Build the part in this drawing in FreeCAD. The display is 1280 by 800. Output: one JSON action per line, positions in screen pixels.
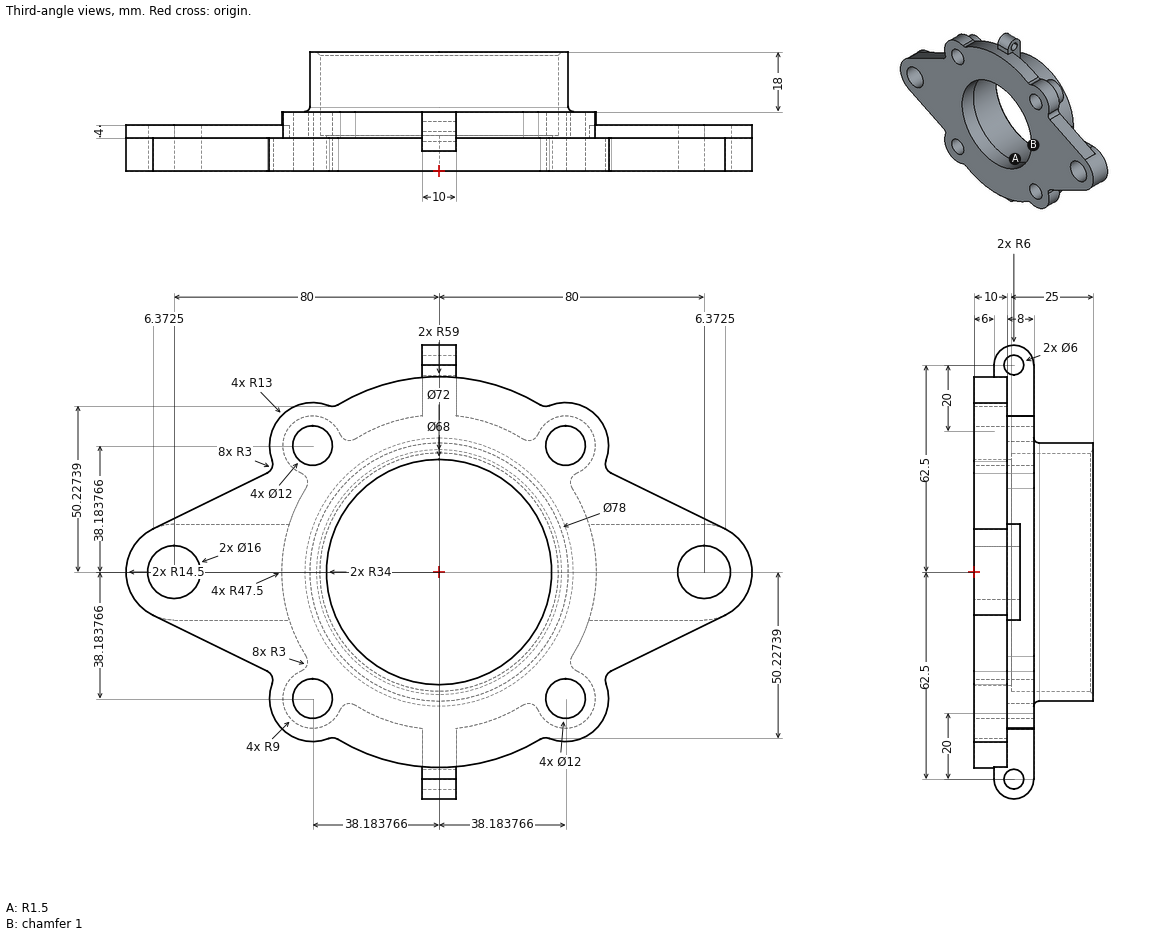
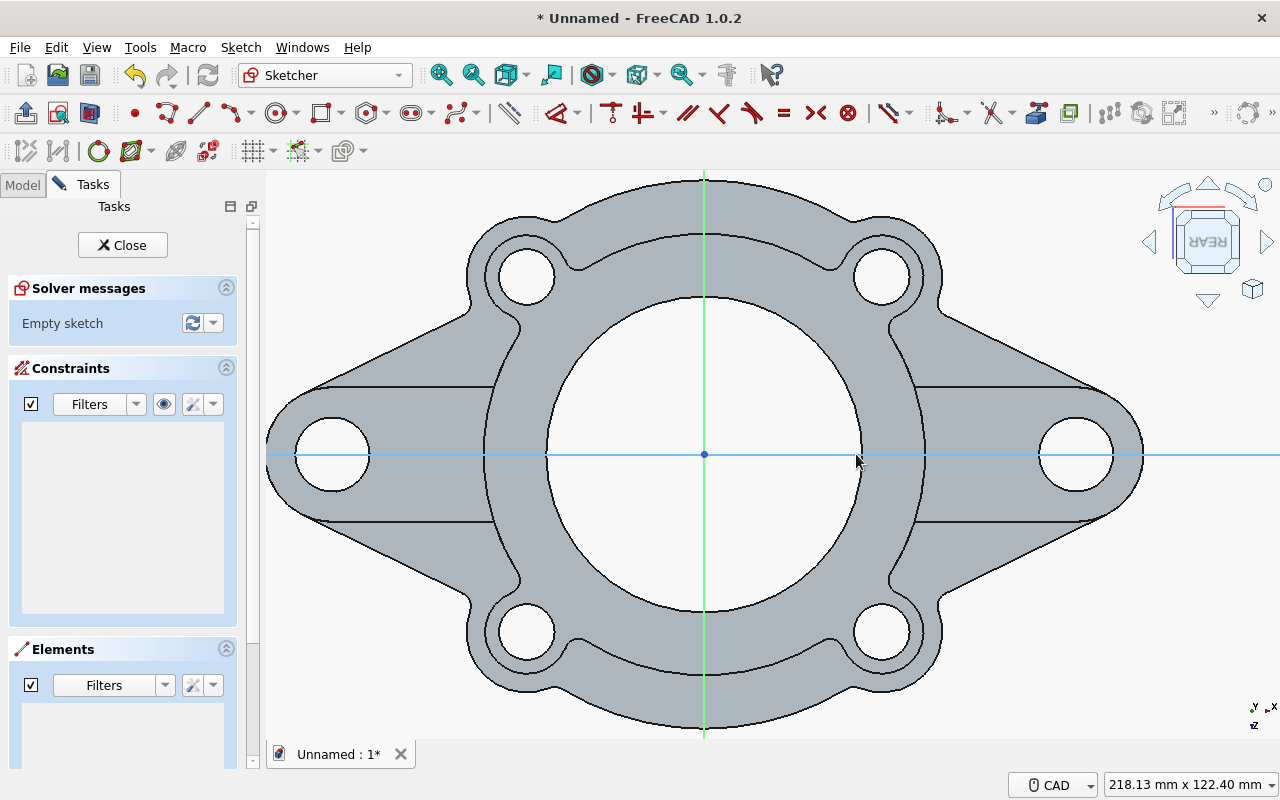
{"action": "left_click", "coordinate": [276, 114]}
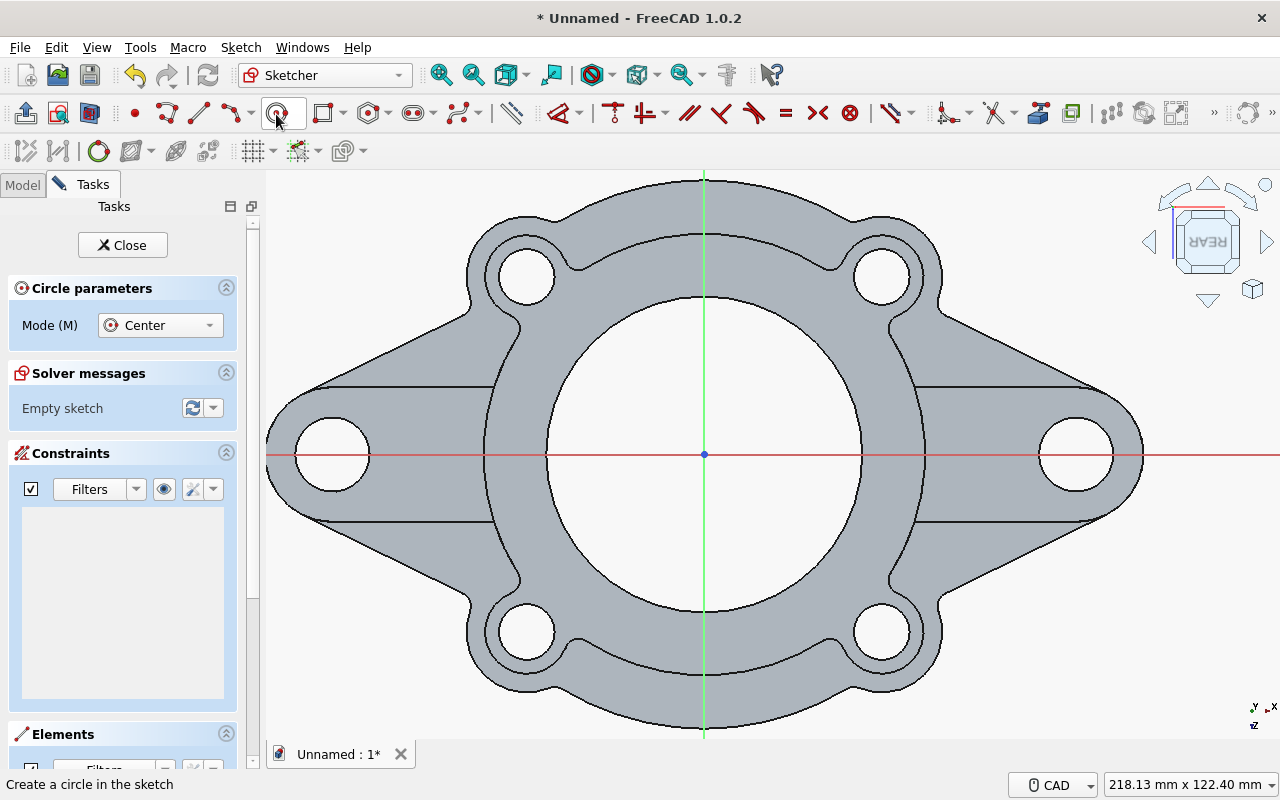
{"action": "left_click", "coordinate": [704, 454]}
{"action": "mouse_move", "coordinate": [832, 326]}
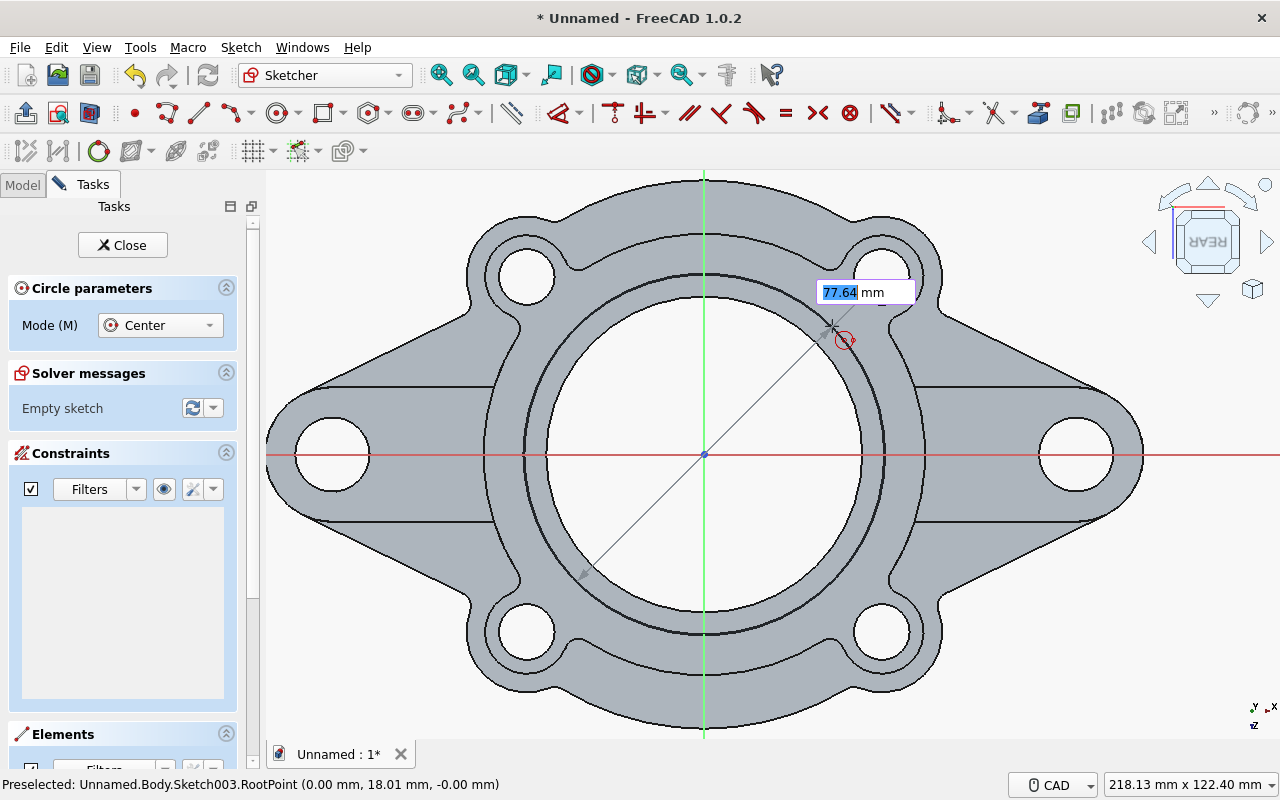
{"action": "type", "text": "78"}
{"action": "key", "text": "Return"}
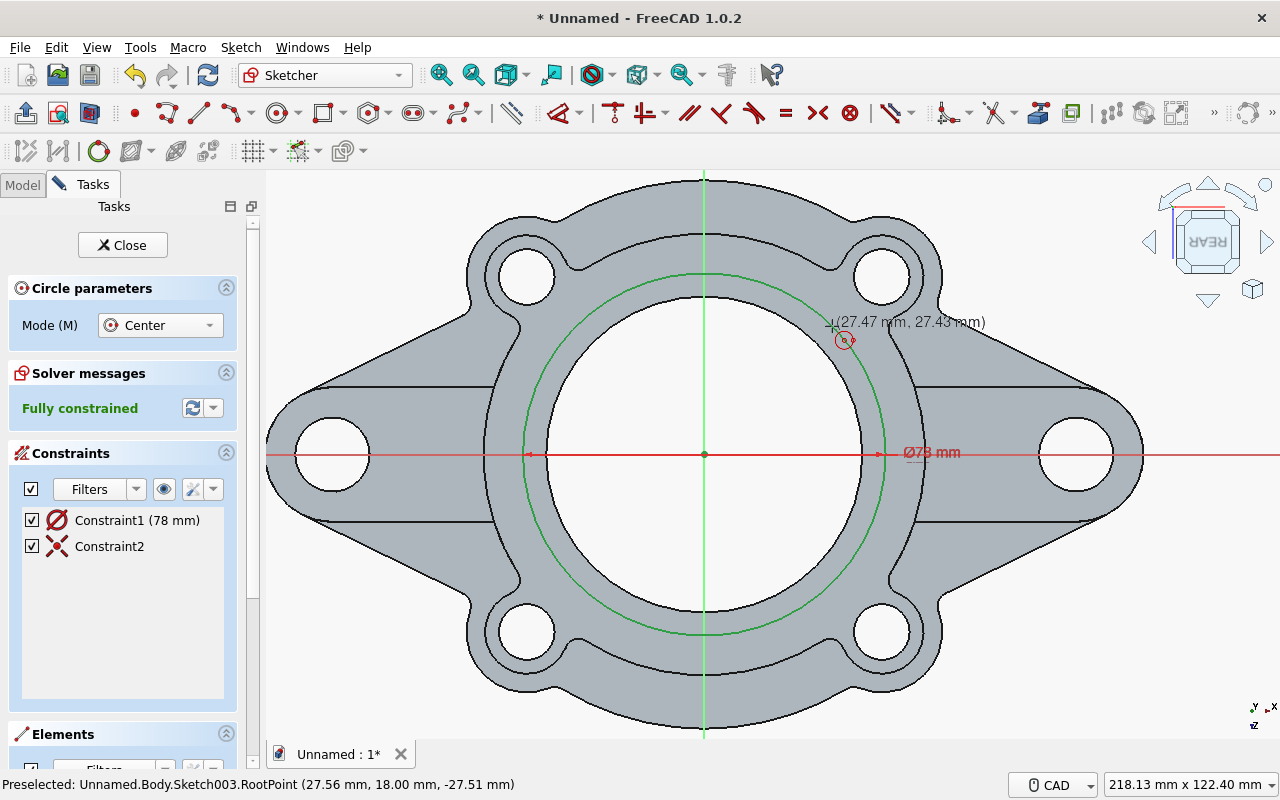
{"action": "left_click", "coordinate": [704, 454]}
{"action": "mouse_move", "coordinate": [816, 343]}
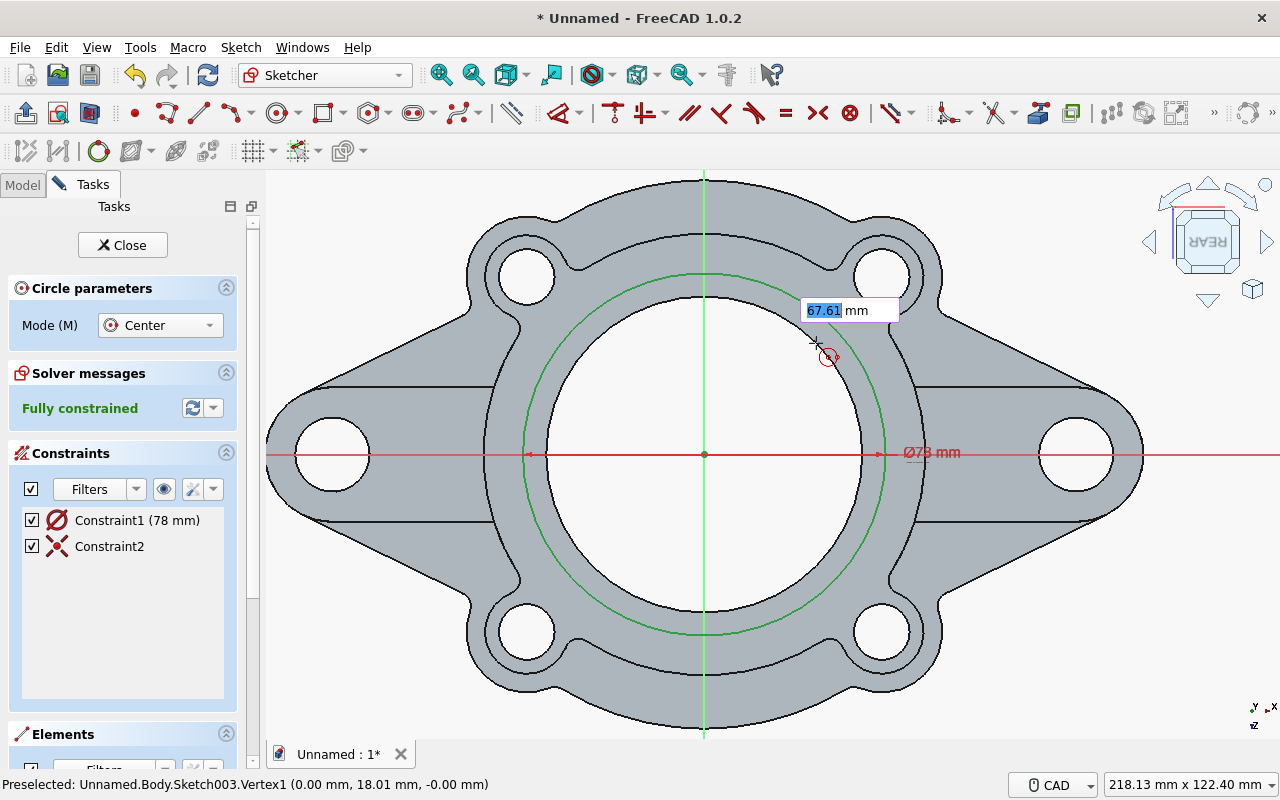
{"action": "type", "text": "68"}
{"action": "key", "text": "Return"}
{"action": "key", "text": "Escape"}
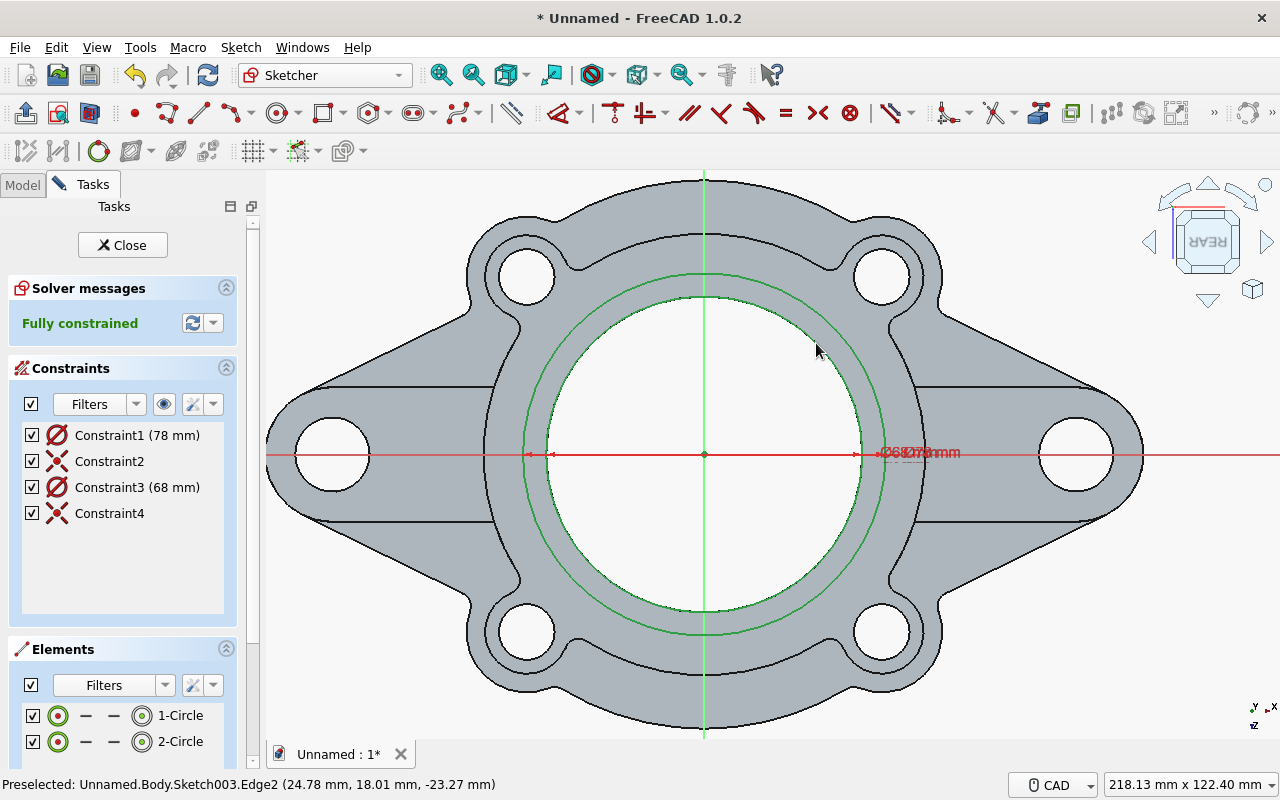
{"action": "left_click", "coordinate": [123, 245]}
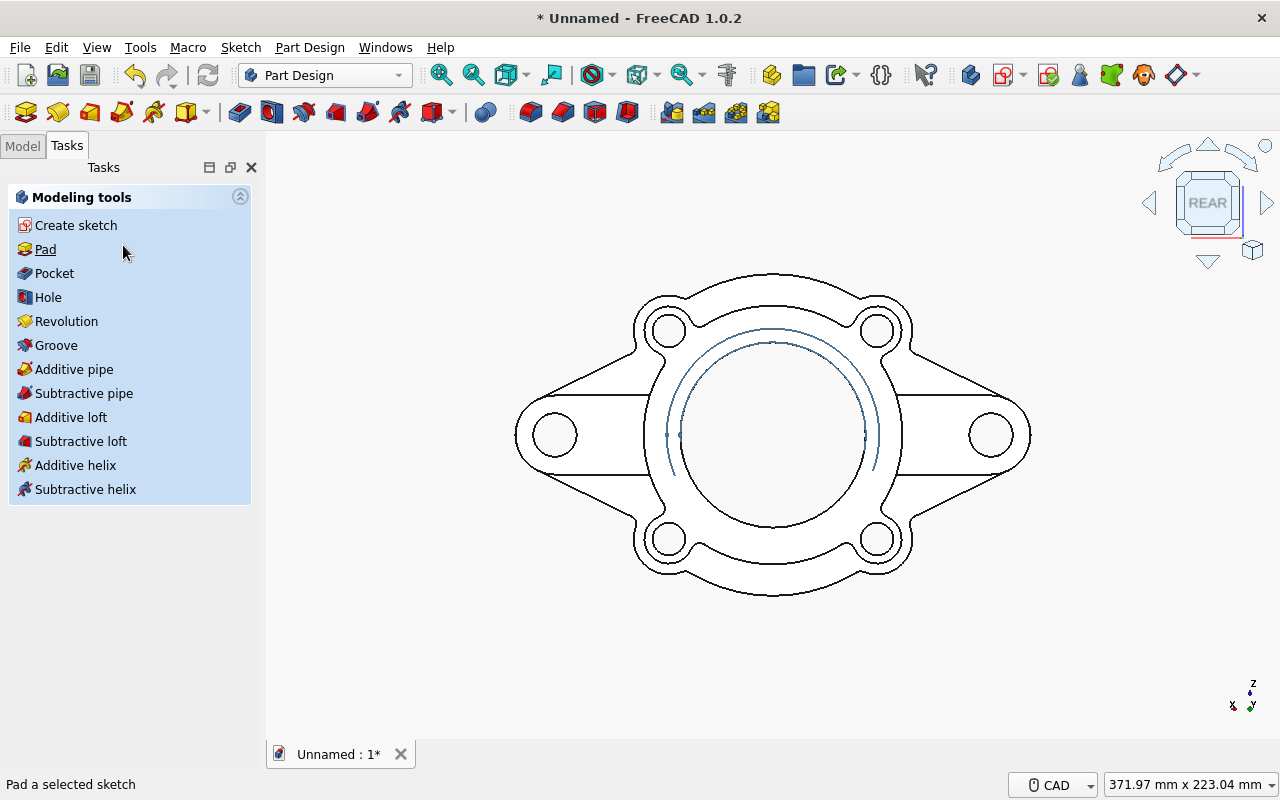
{"action": "left_click", "coordinate": [26, 112]}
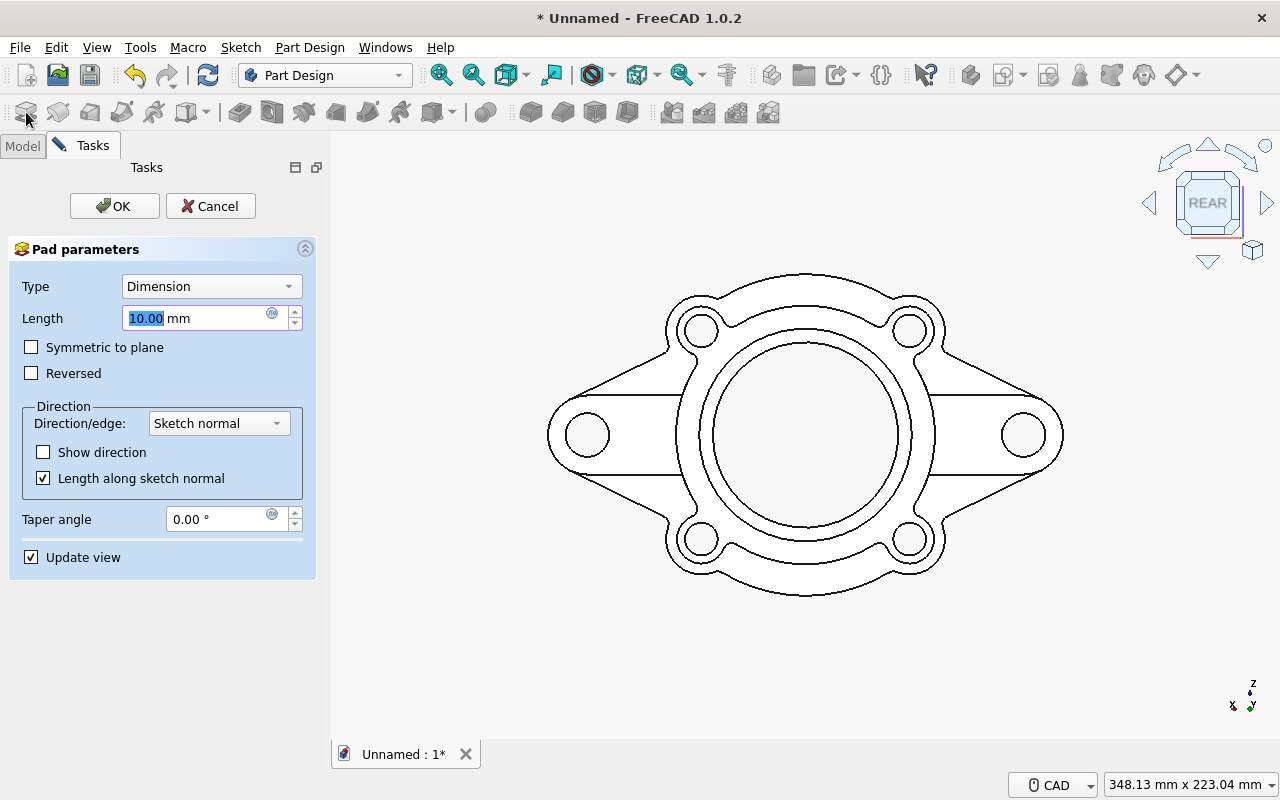
{"action": "type", "text": "18"}
{"action": "key", "text": "Tab"}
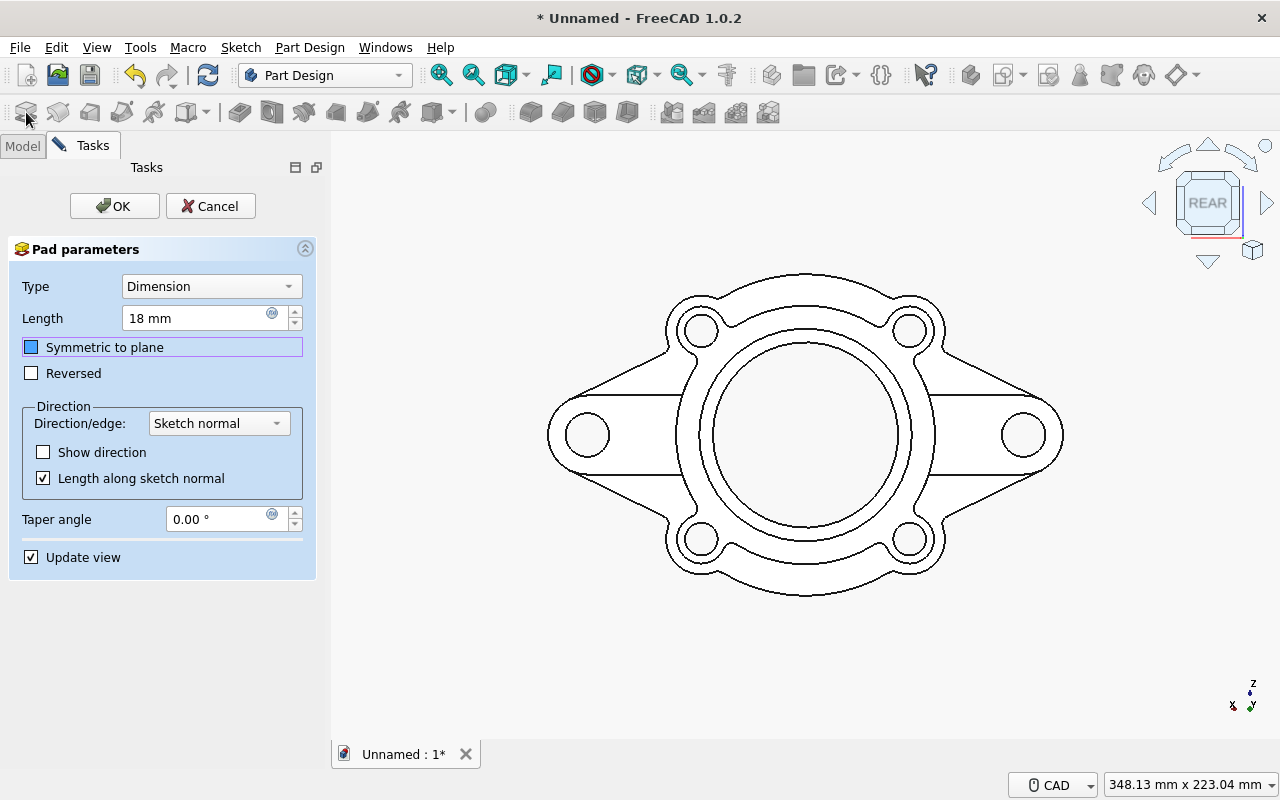
{"action": "left_click", "coordinate": [115, 206]}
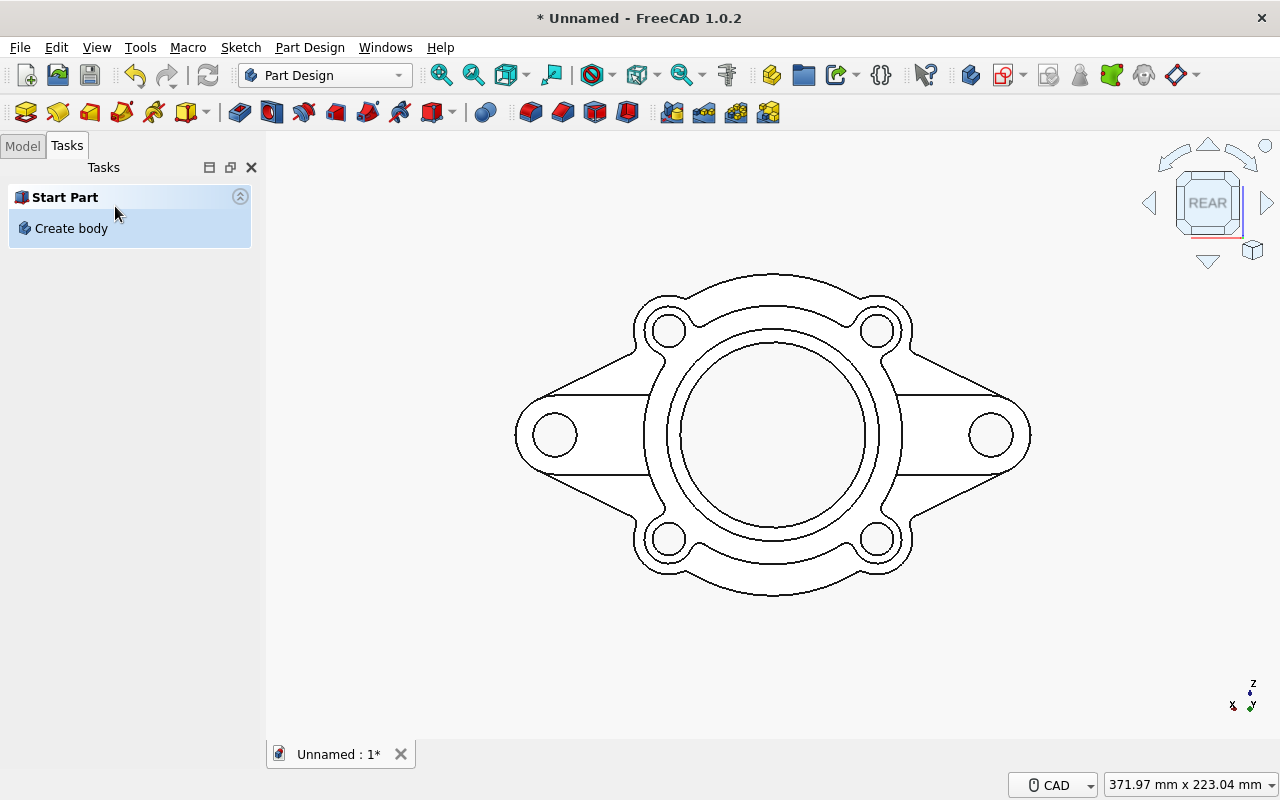
{"action": "key", "text": "0"}